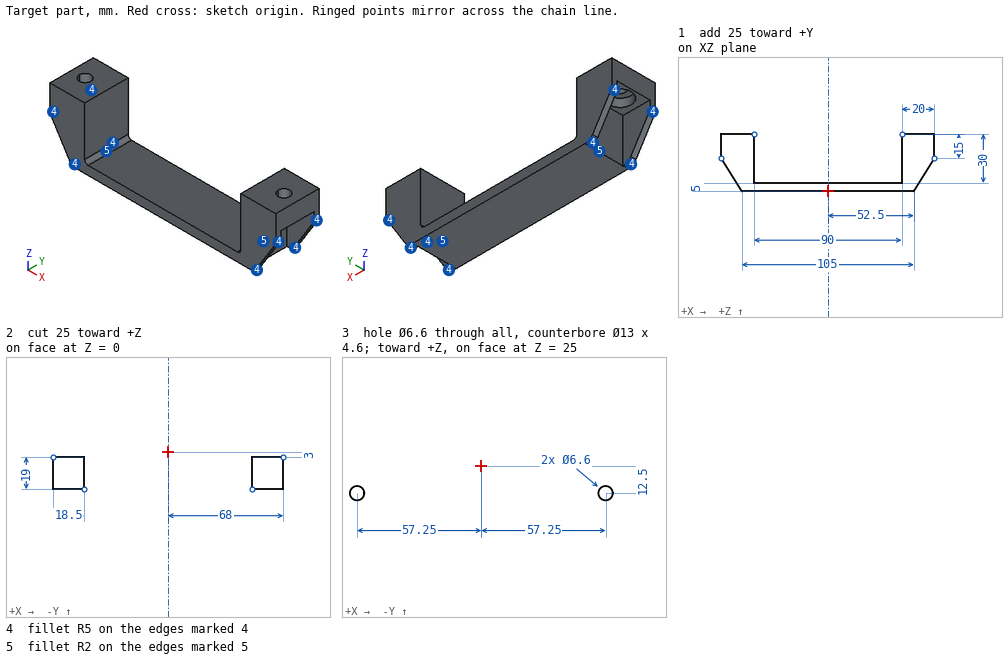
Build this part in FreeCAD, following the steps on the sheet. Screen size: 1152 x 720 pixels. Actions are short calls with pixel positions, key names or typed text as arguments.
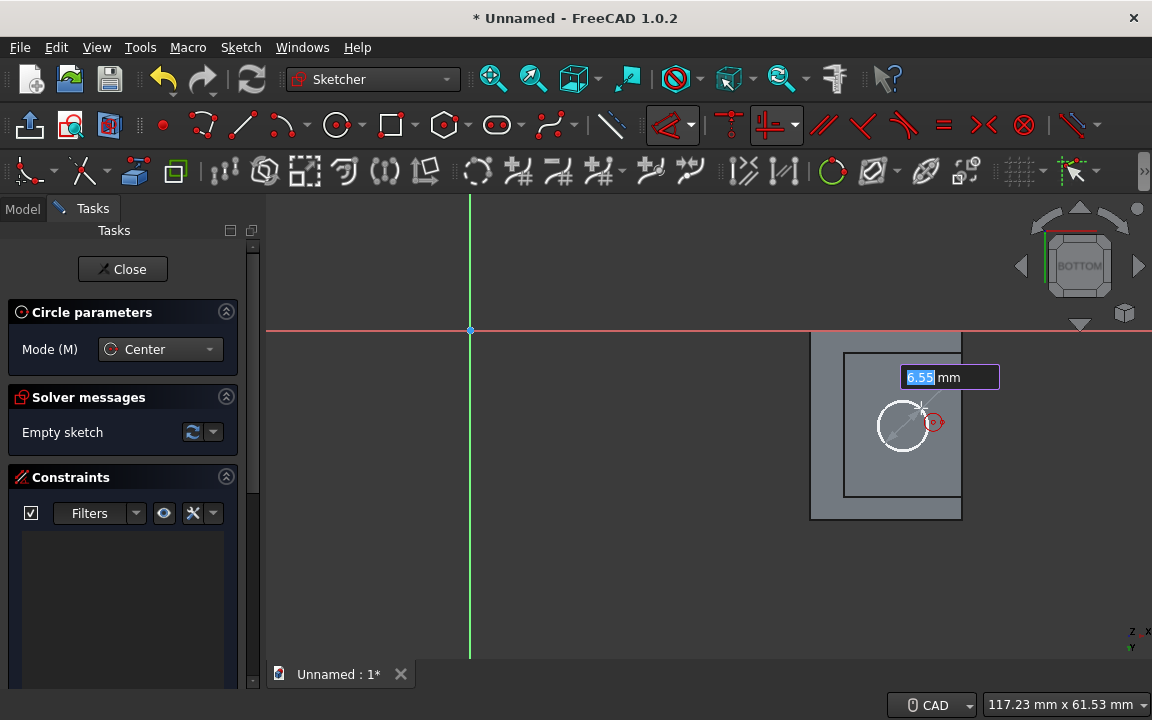
text(6.6)
key(Return)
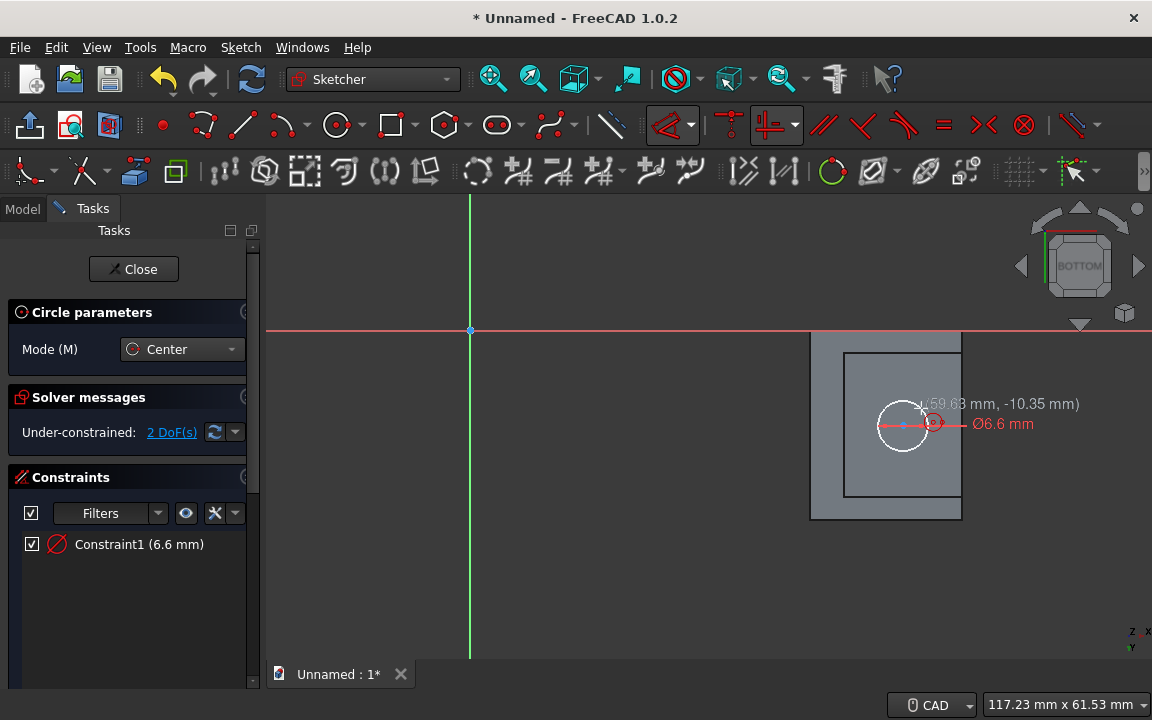
scroll(847, 470, down, 3)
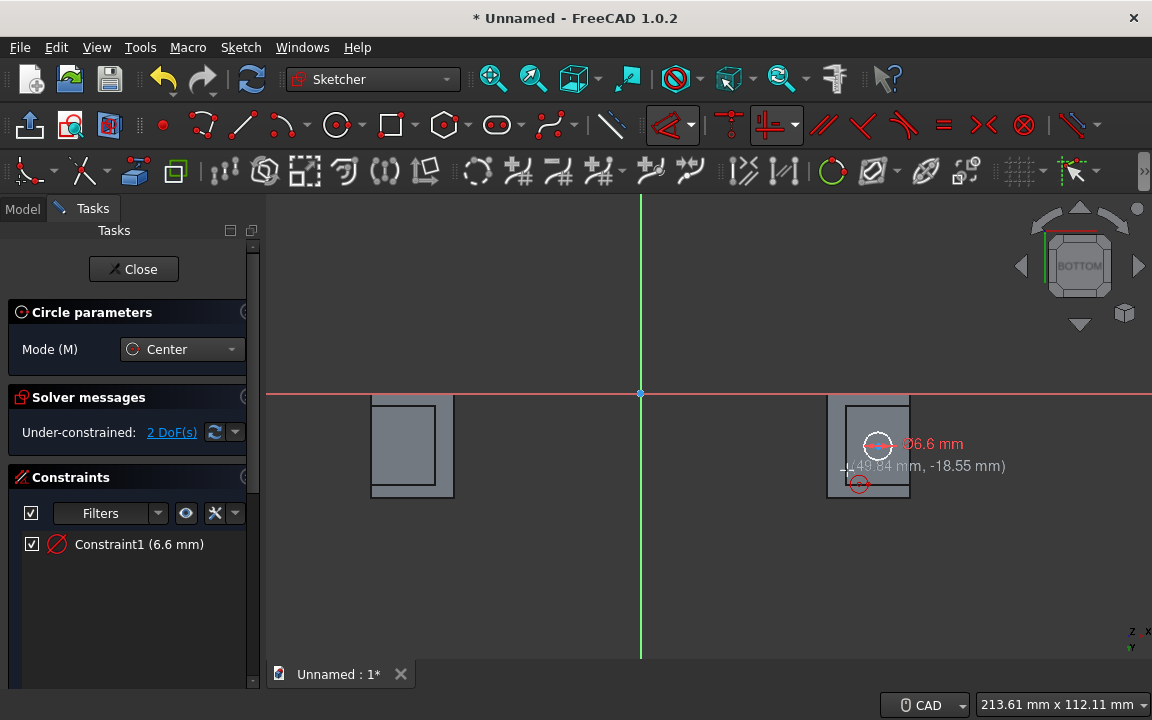
scroll(403, 446, up, 3)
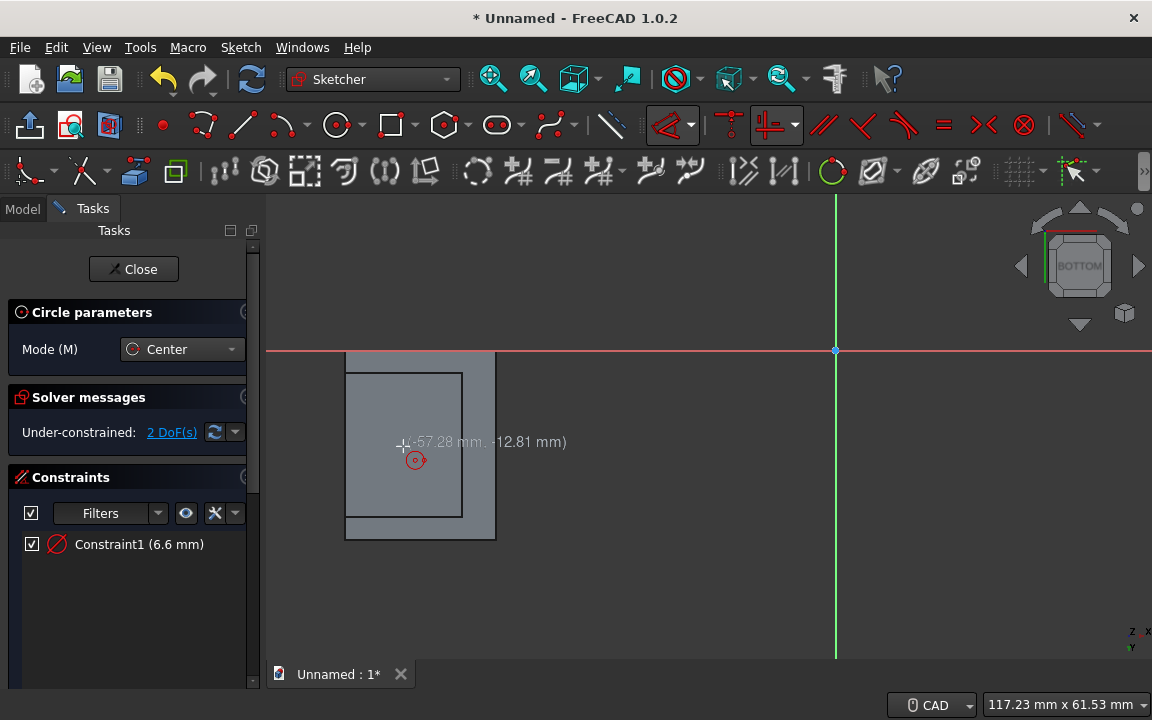
click(403, 445)
move(421, 427)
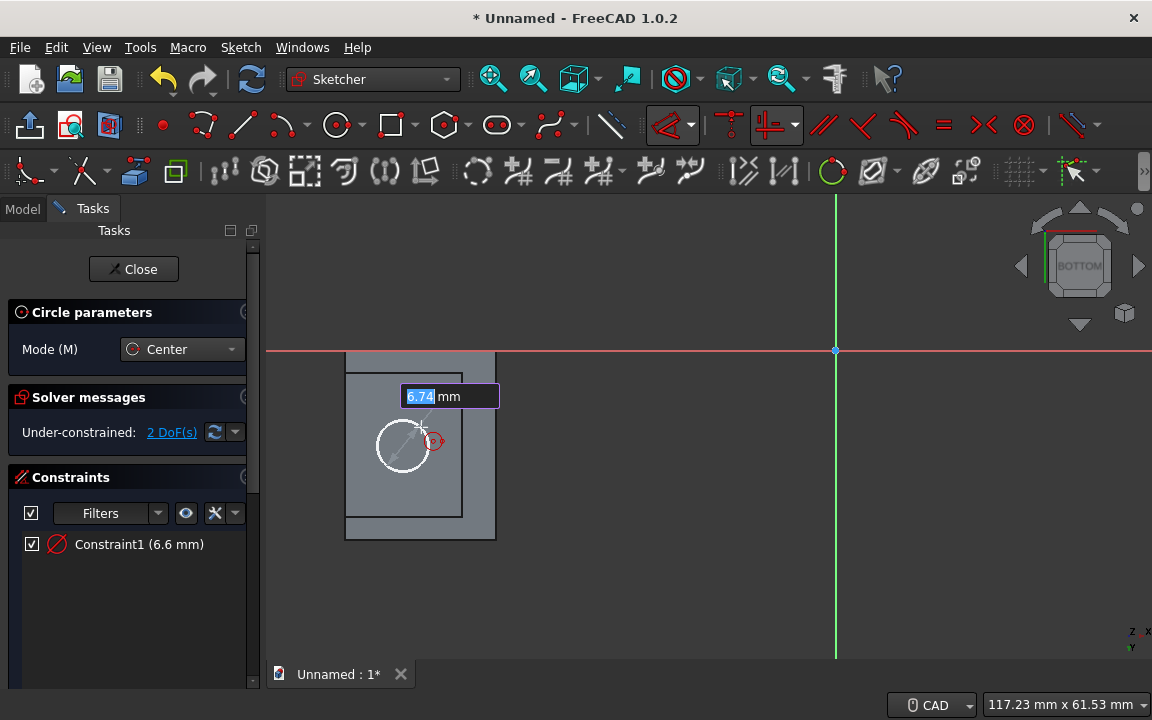
text(6.6)
key(Return)
key(Escape)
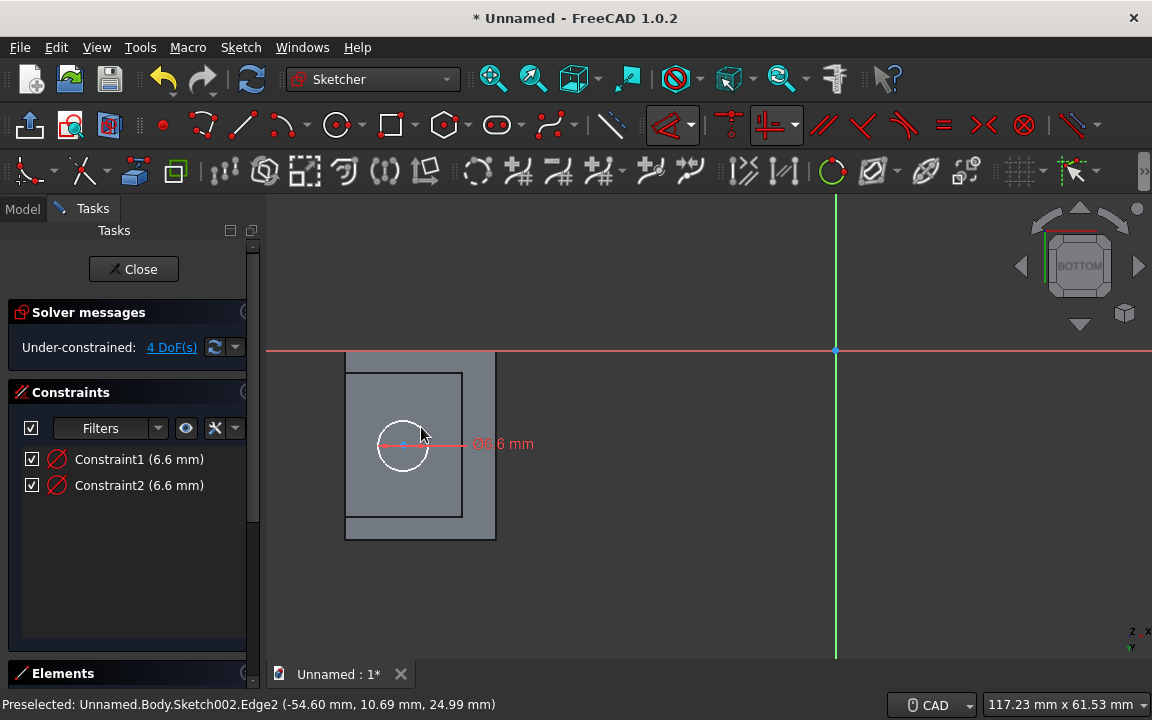
scroll(403, 446, down, 3)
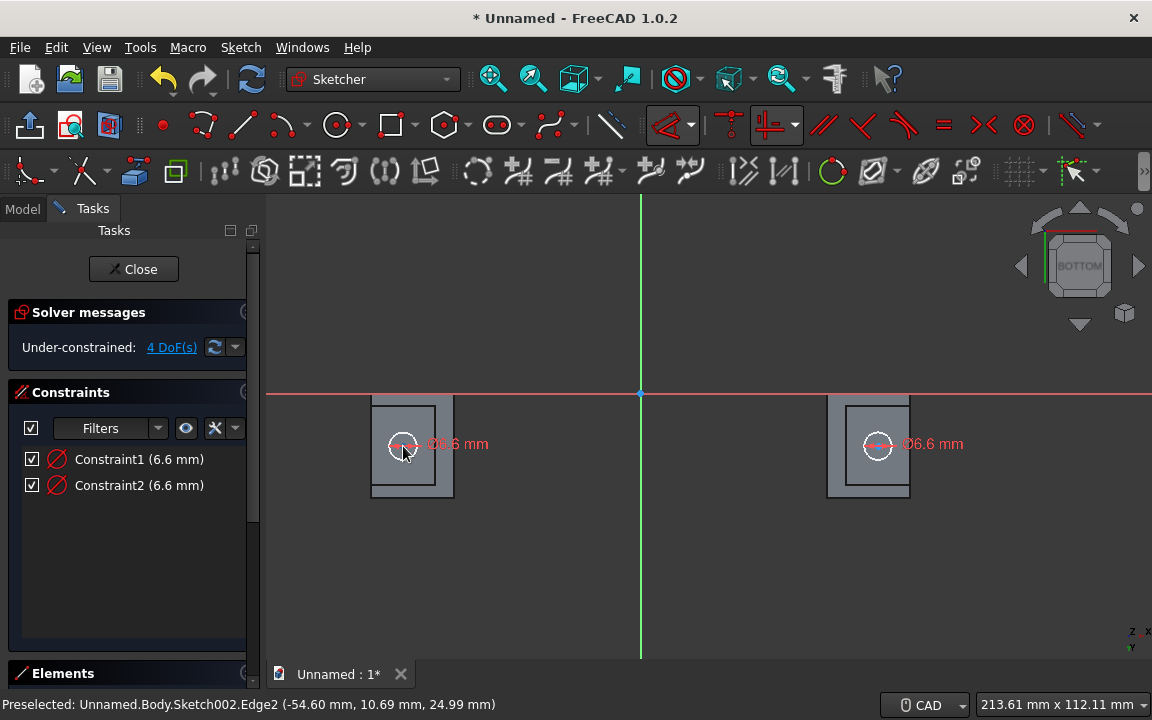
click(878, 446)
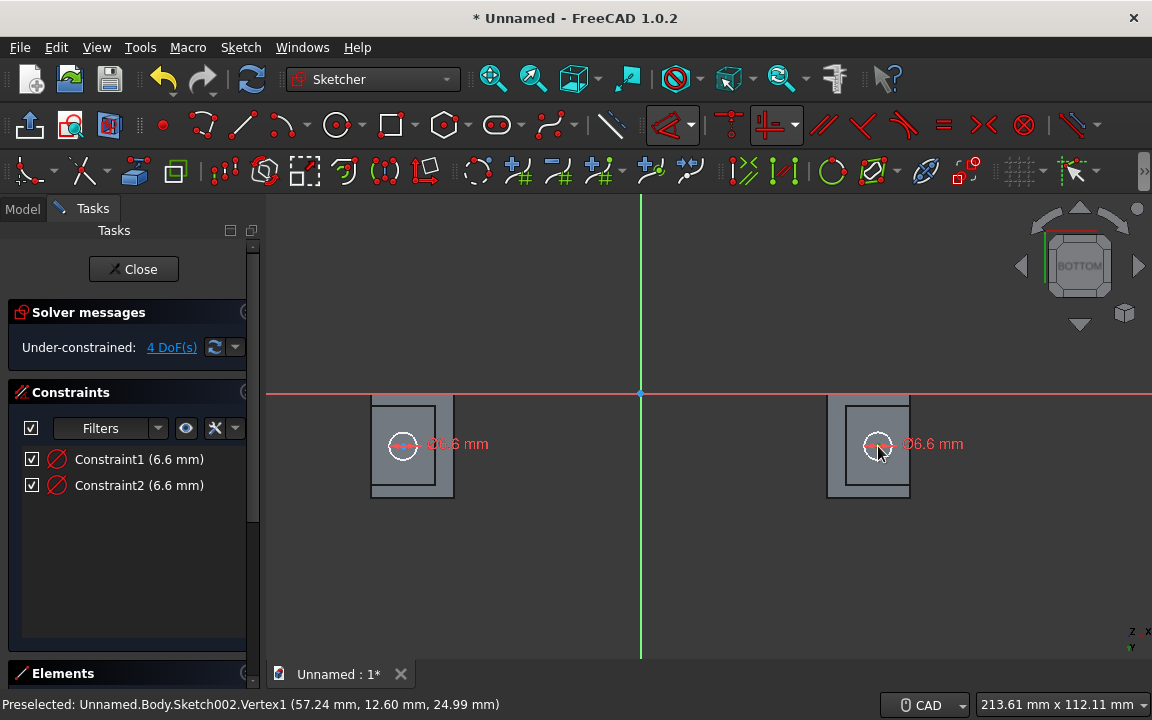
click(403, 446)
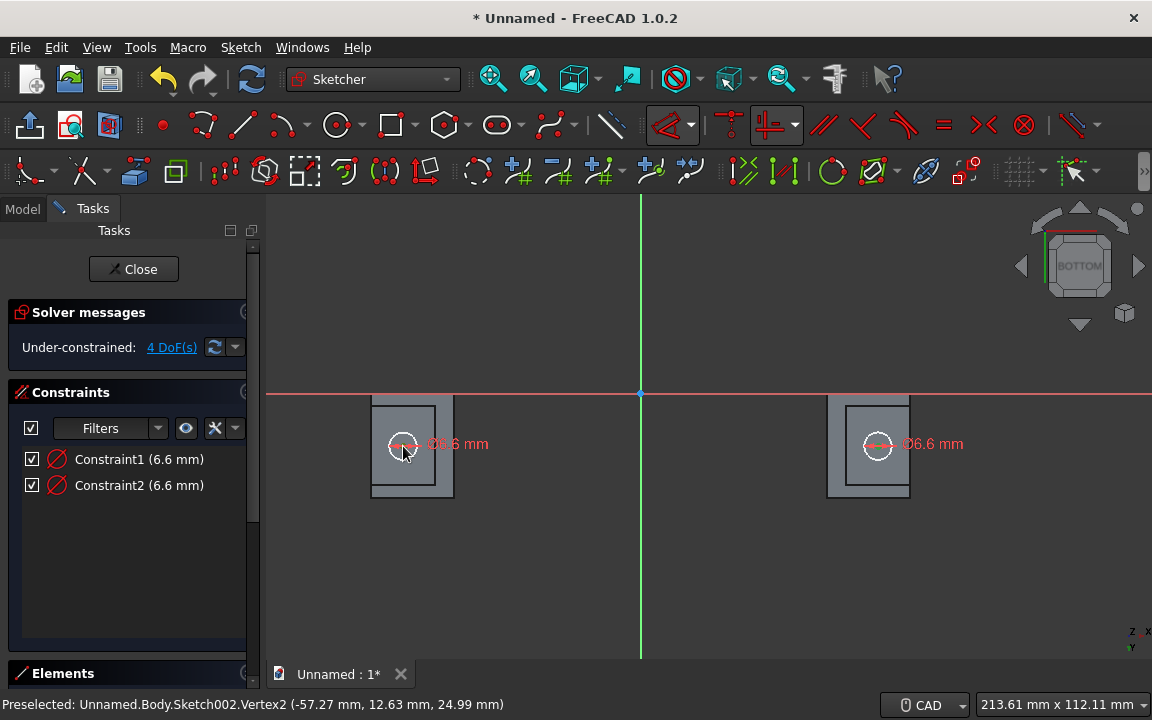
click(798, 126)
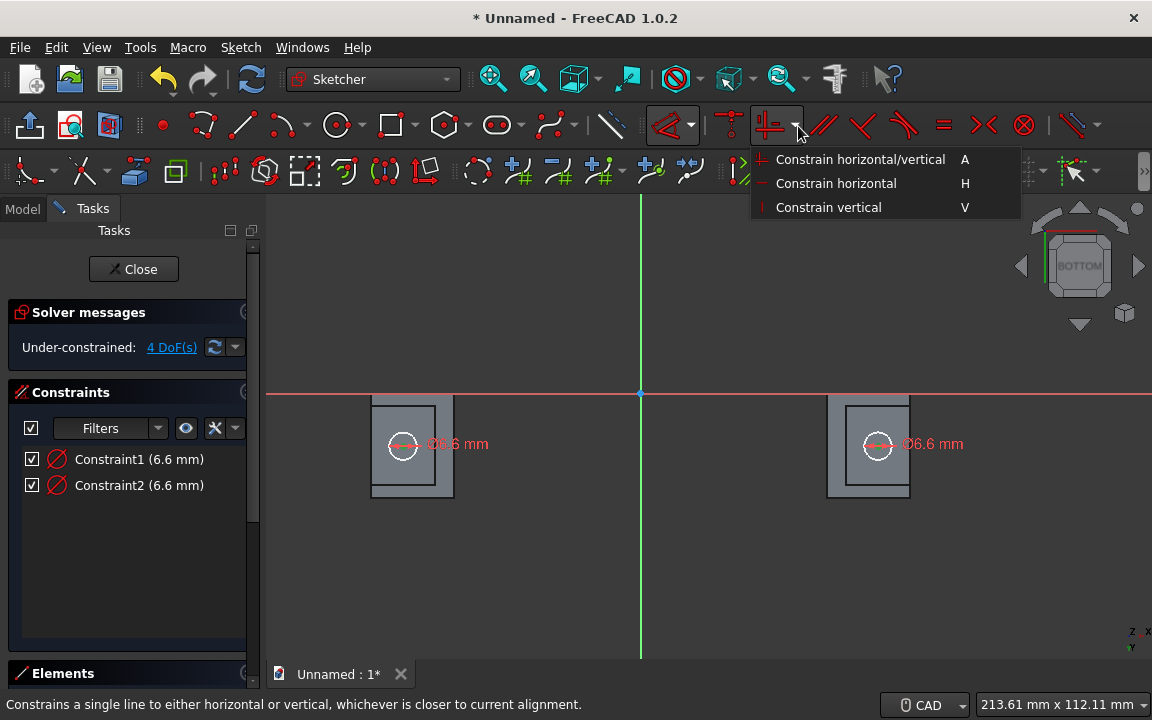
click(886, 183)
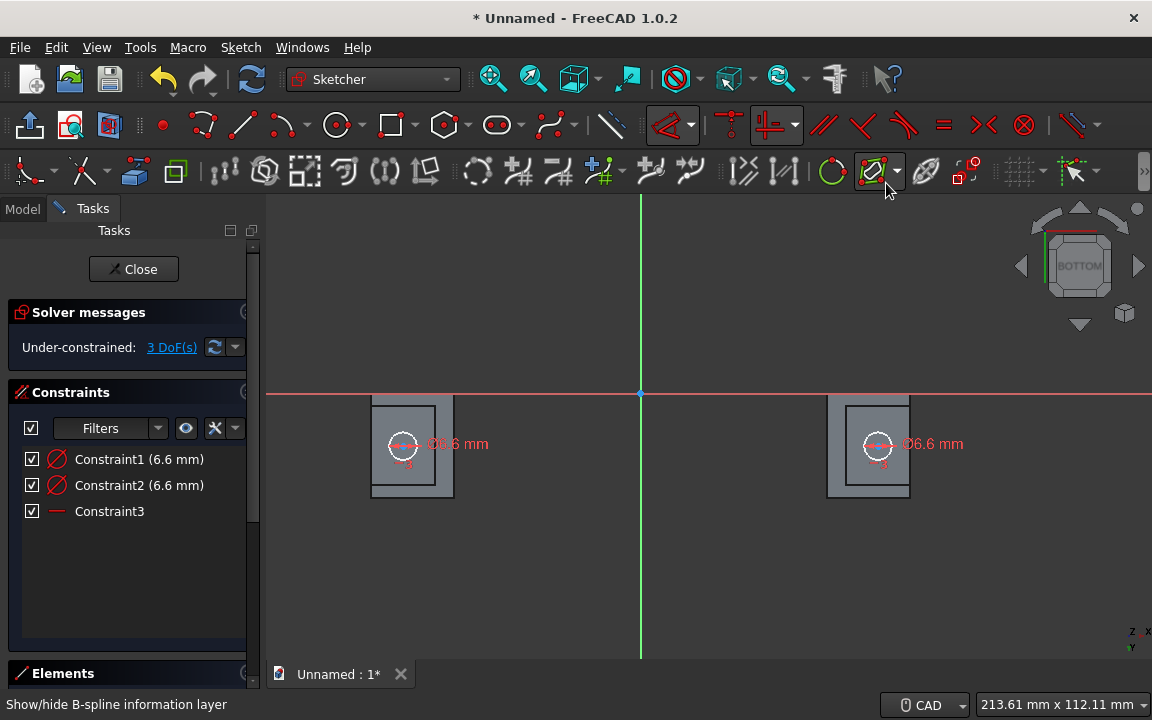
click(878, 446)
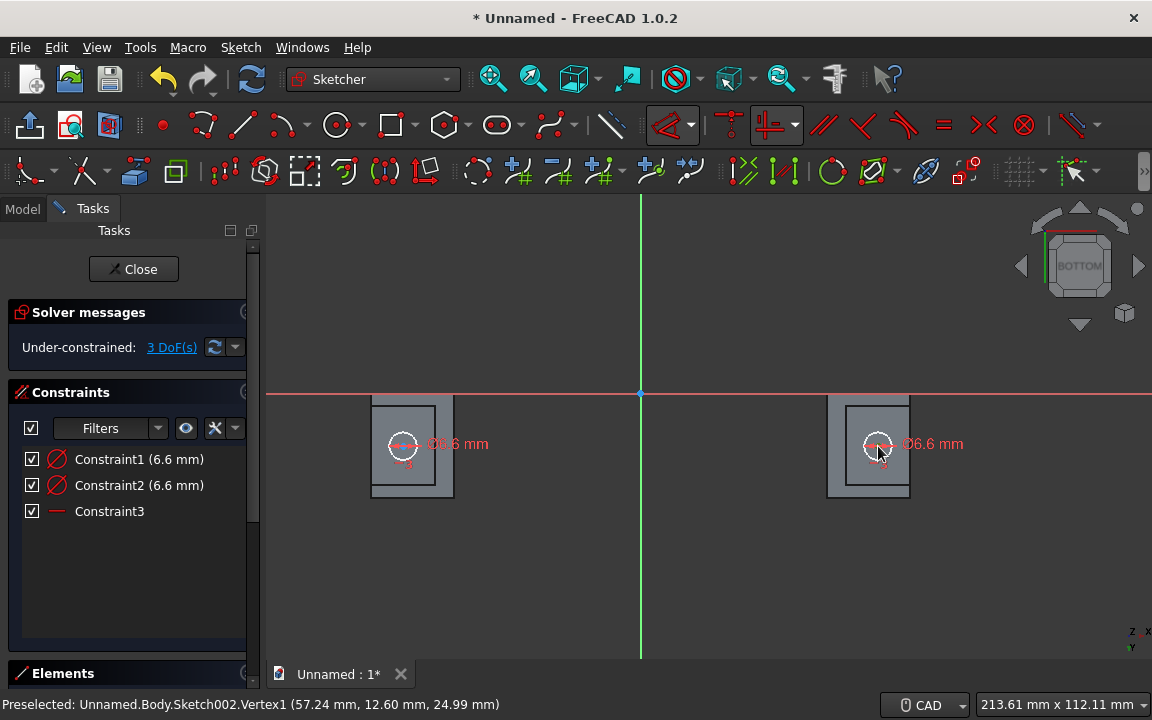
click(694, 126)